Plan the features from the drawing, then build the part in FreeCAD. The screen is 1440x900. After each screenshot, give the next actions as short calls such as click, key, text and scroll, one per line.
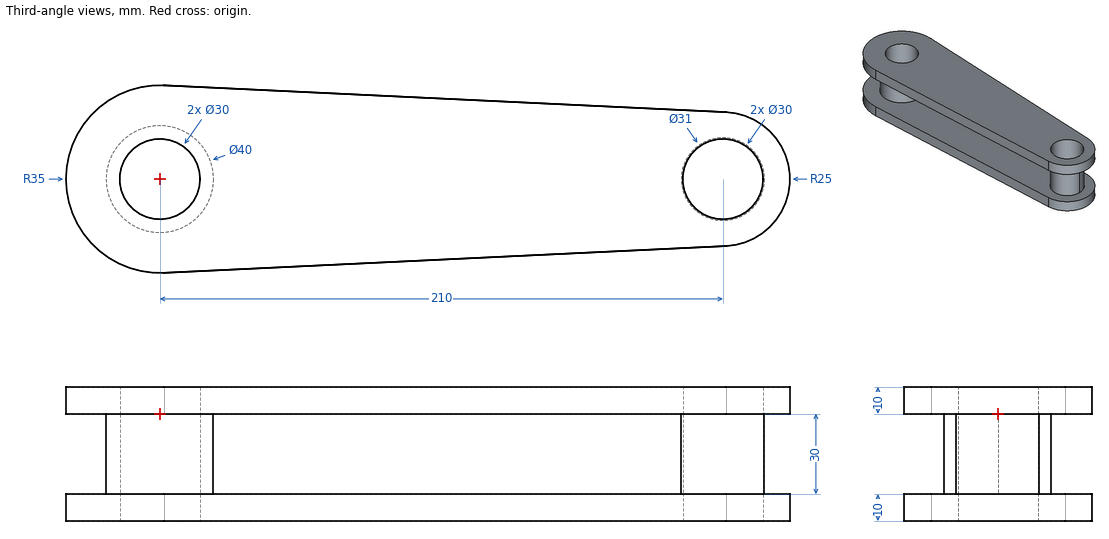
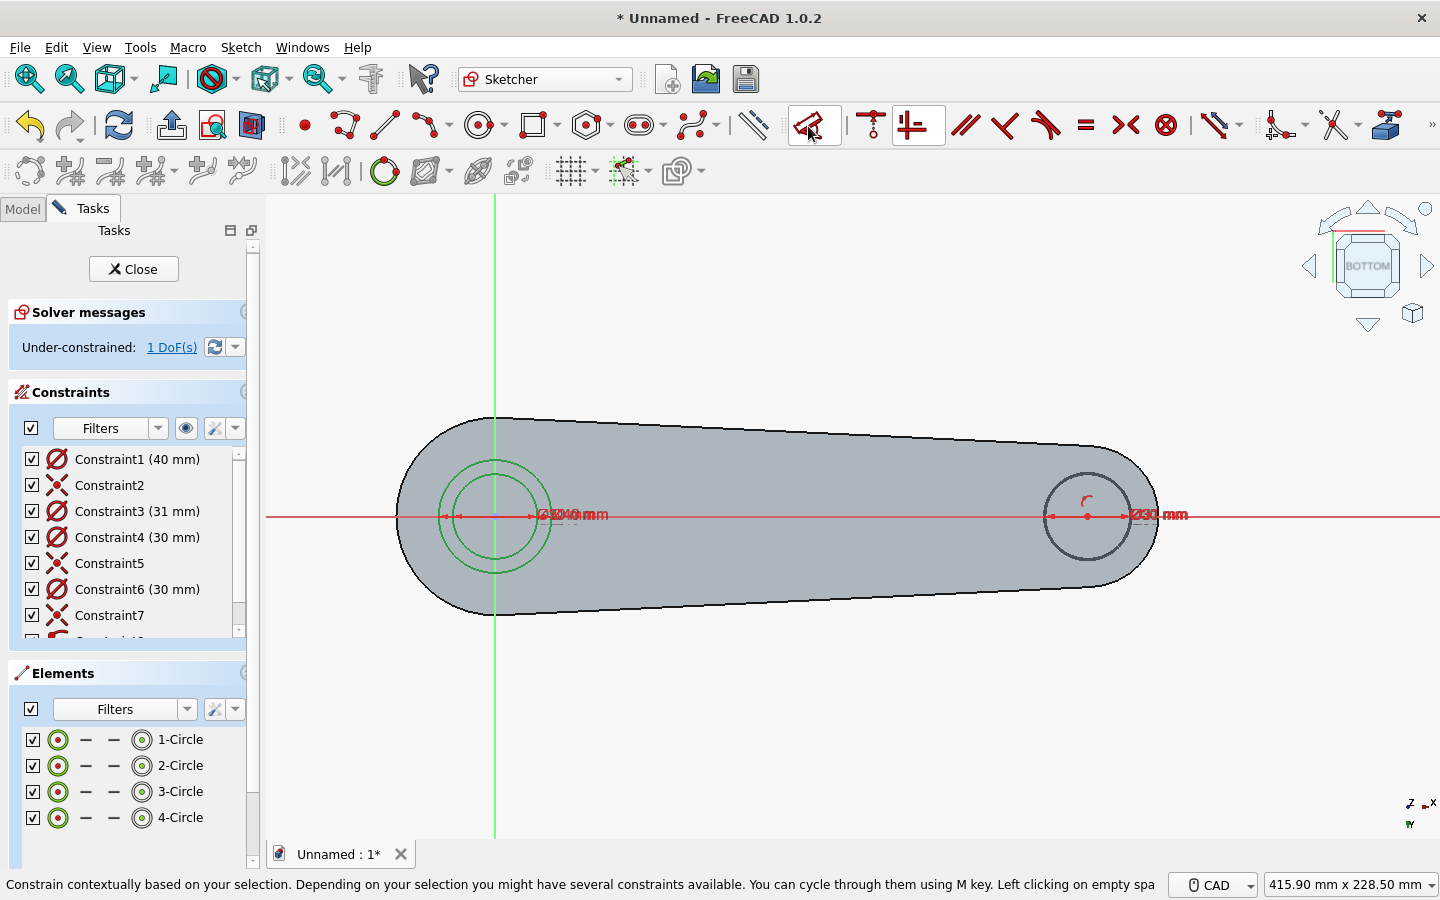
click(1088, 517)
click(791, 551)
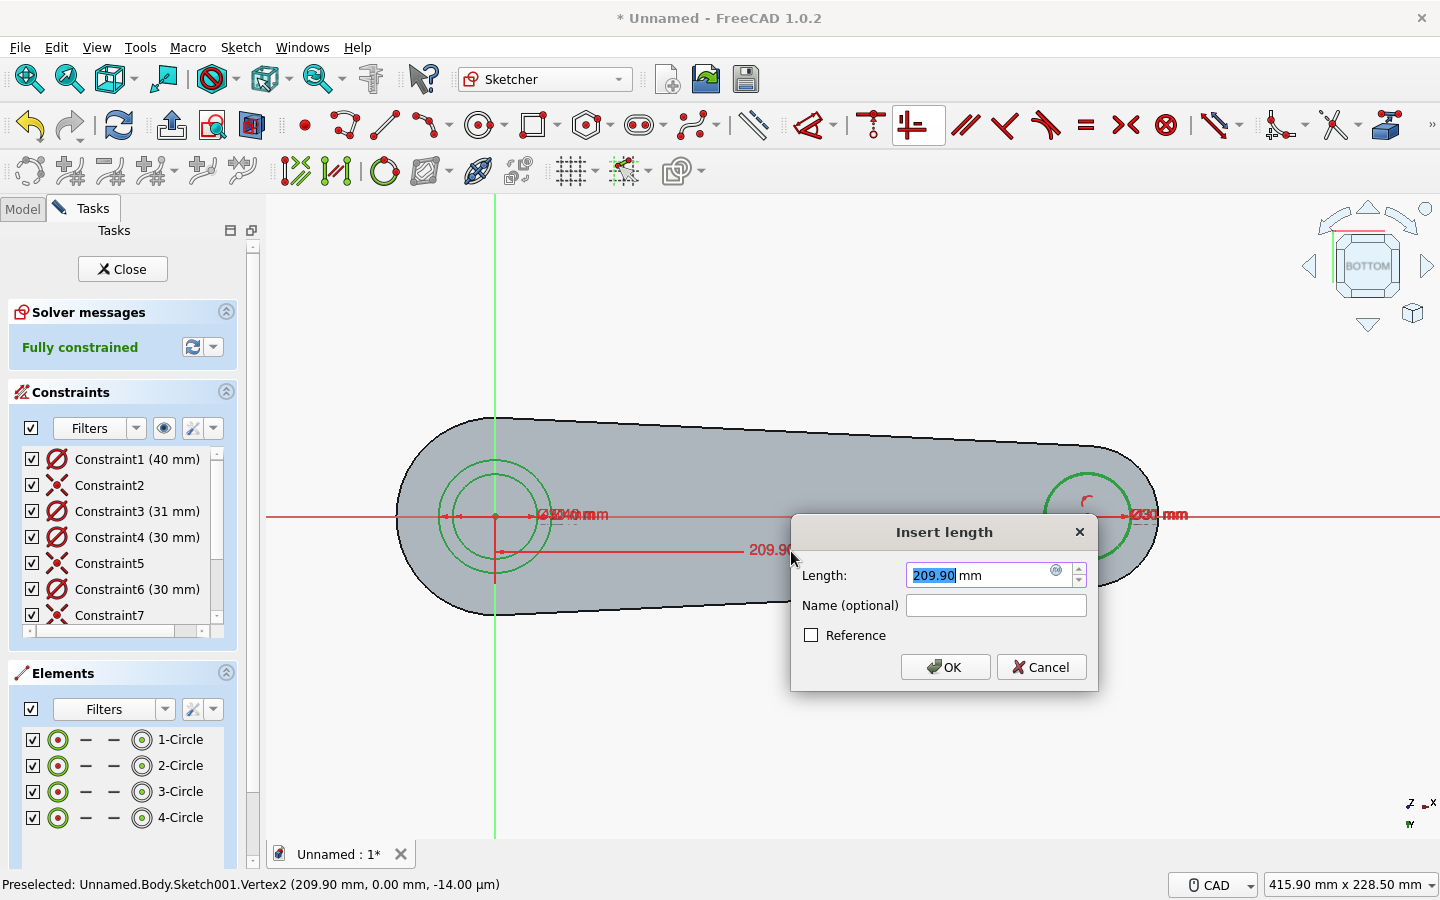
text(210)
key(Return)
key(Escape)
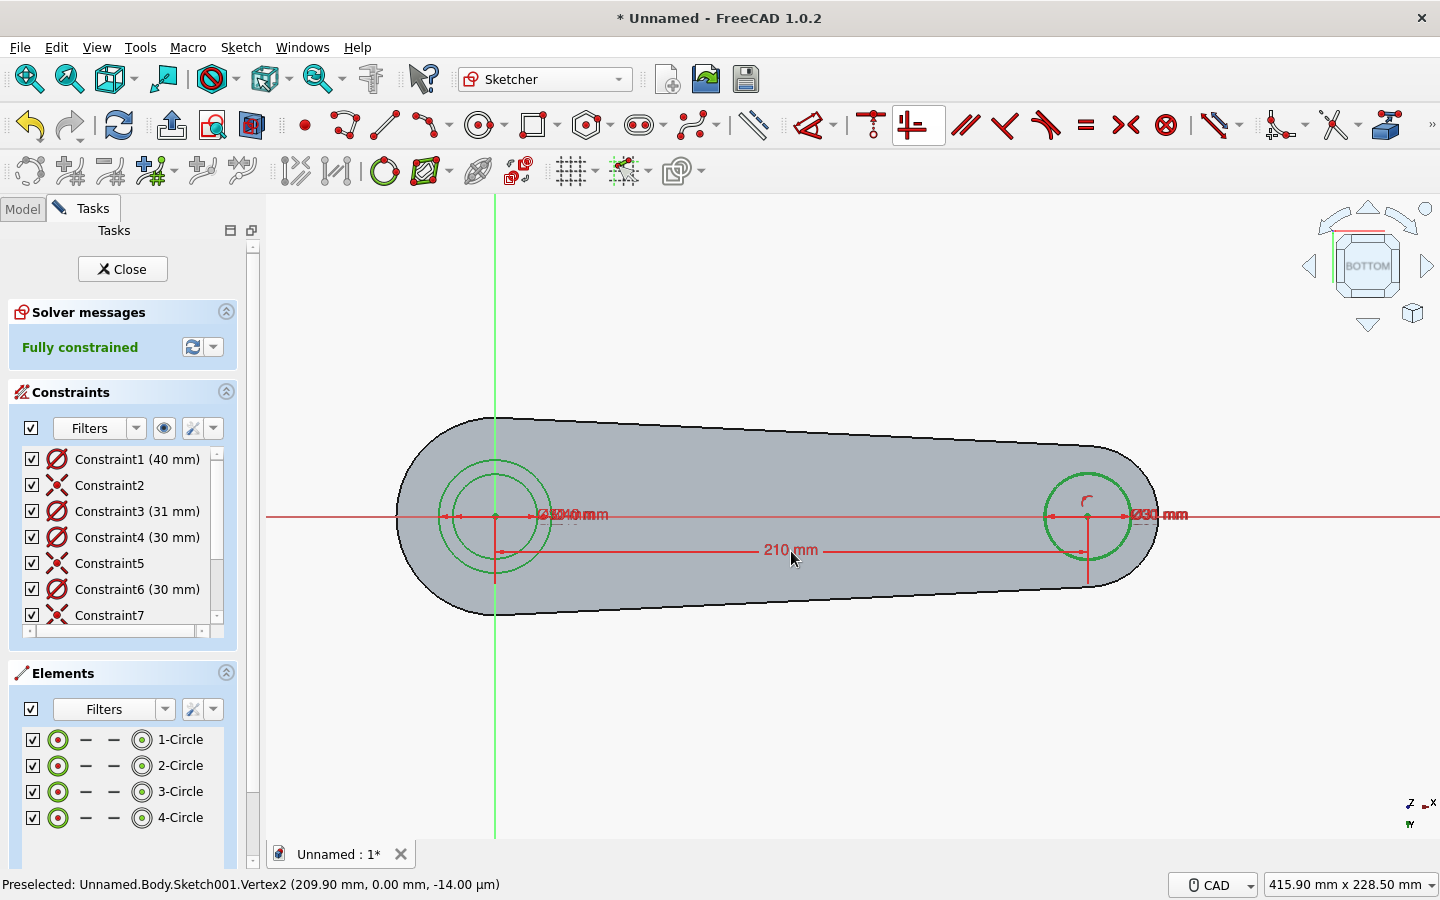
click(123, 269)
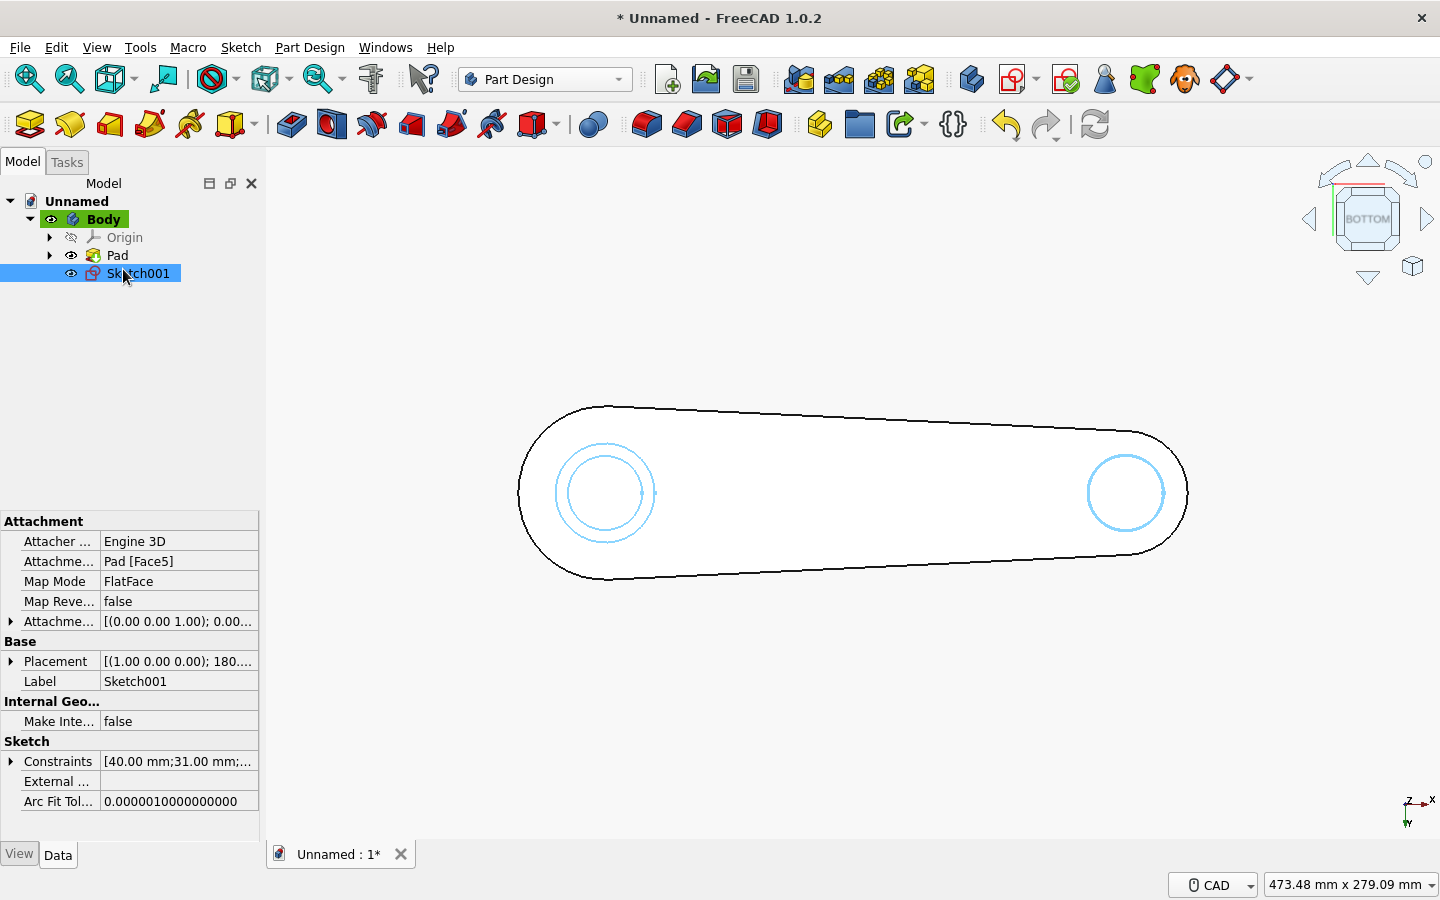
click(30, 124)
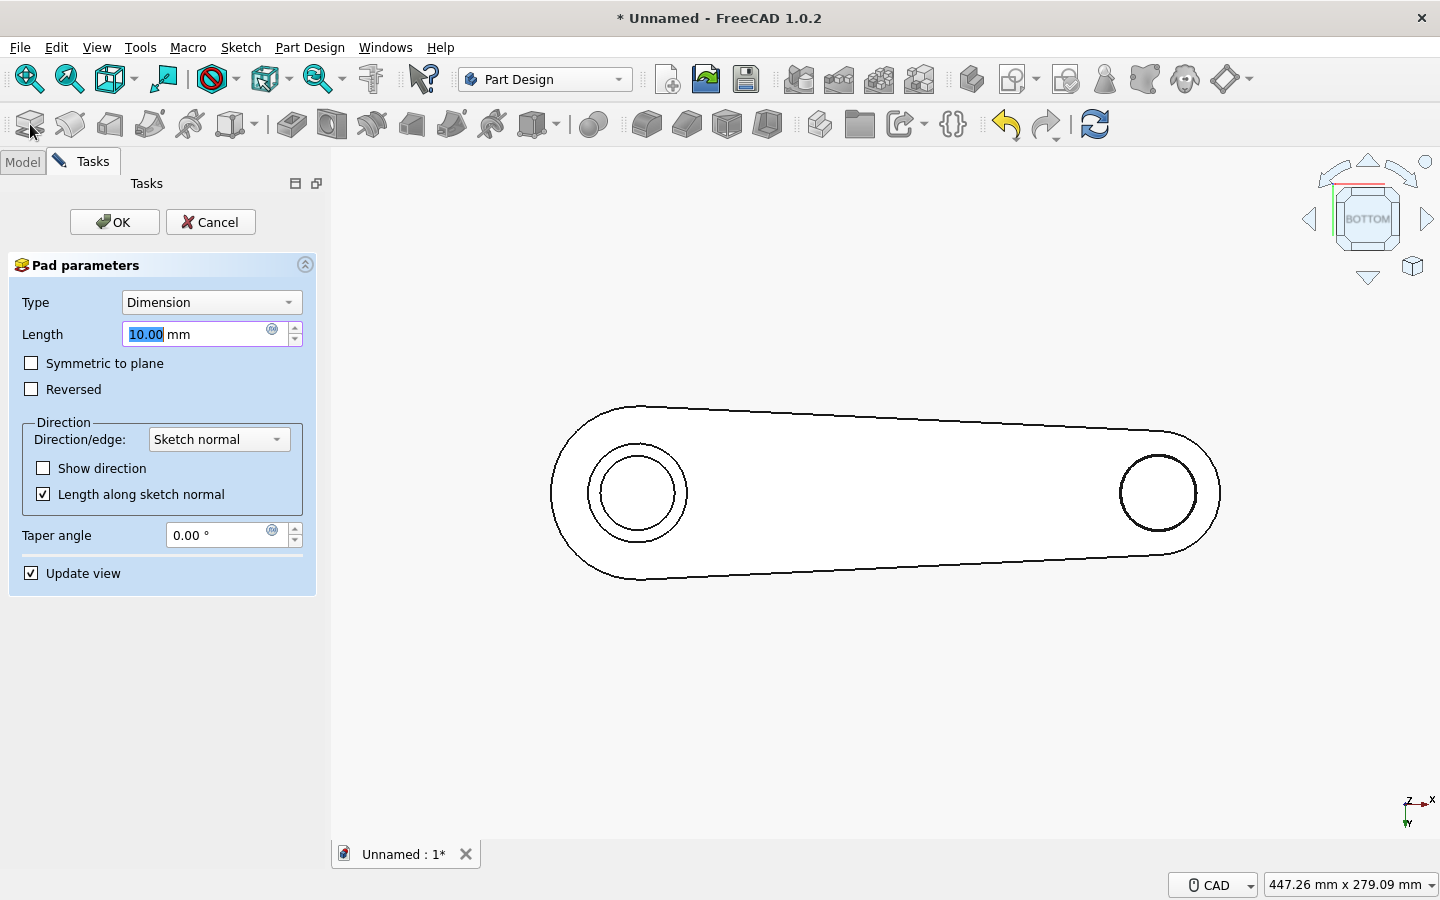
text(30)
key(Tab)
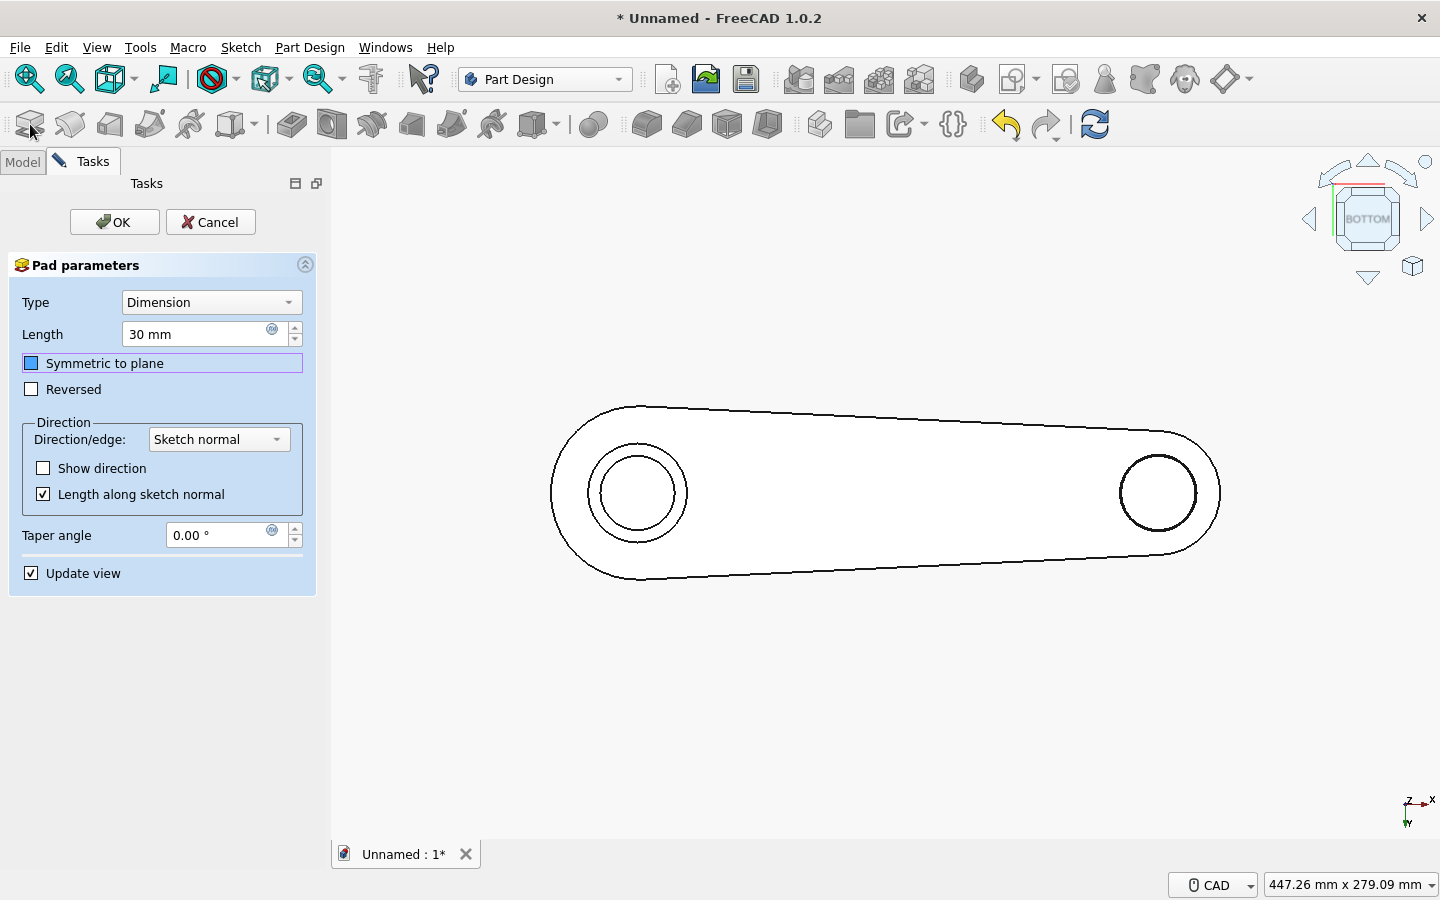
click(115, 222)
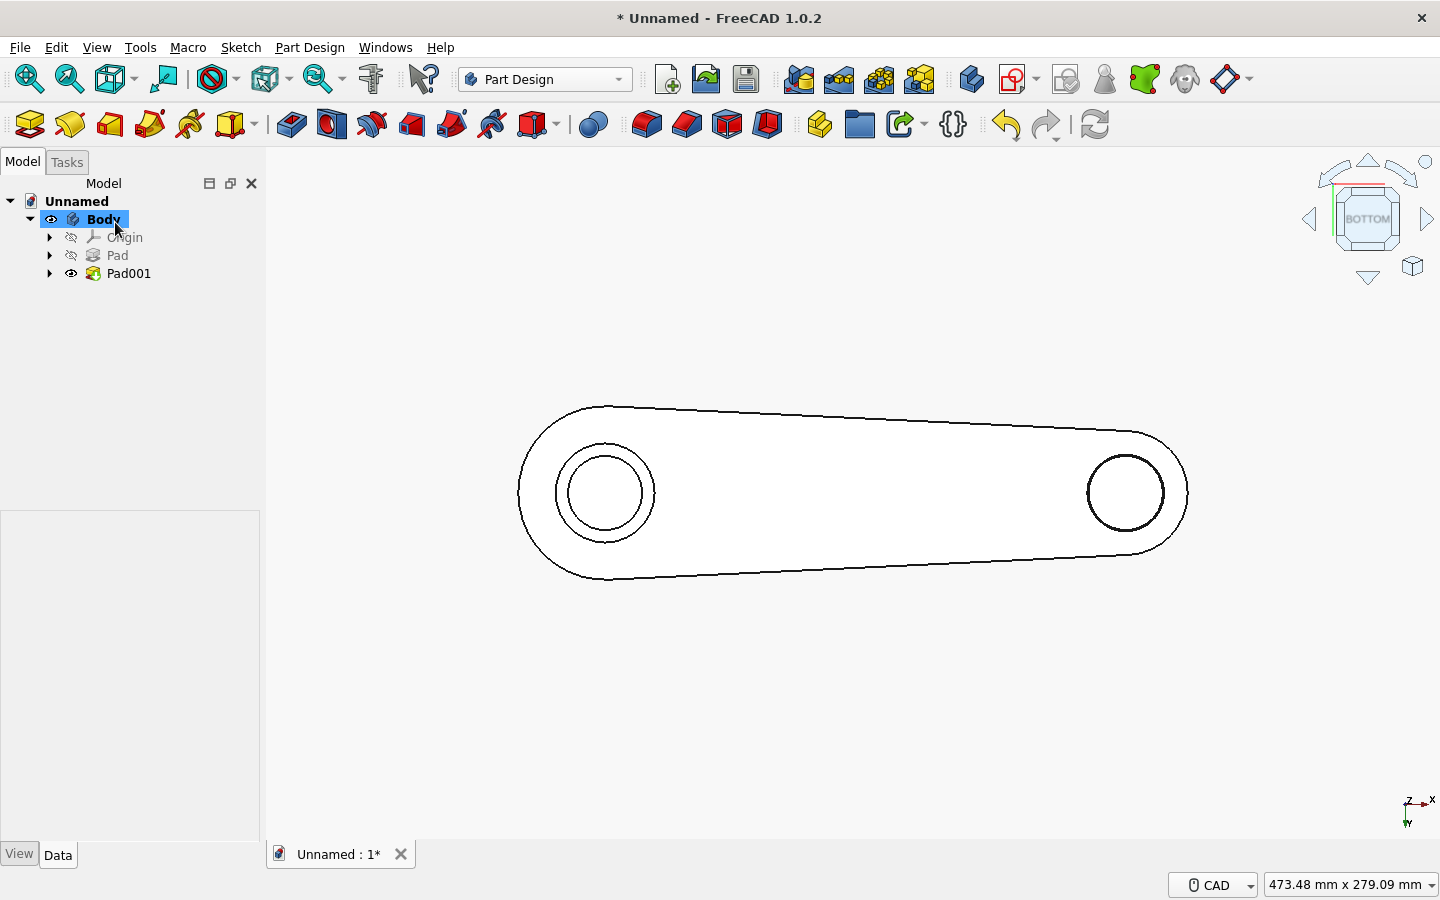
click(50, 237)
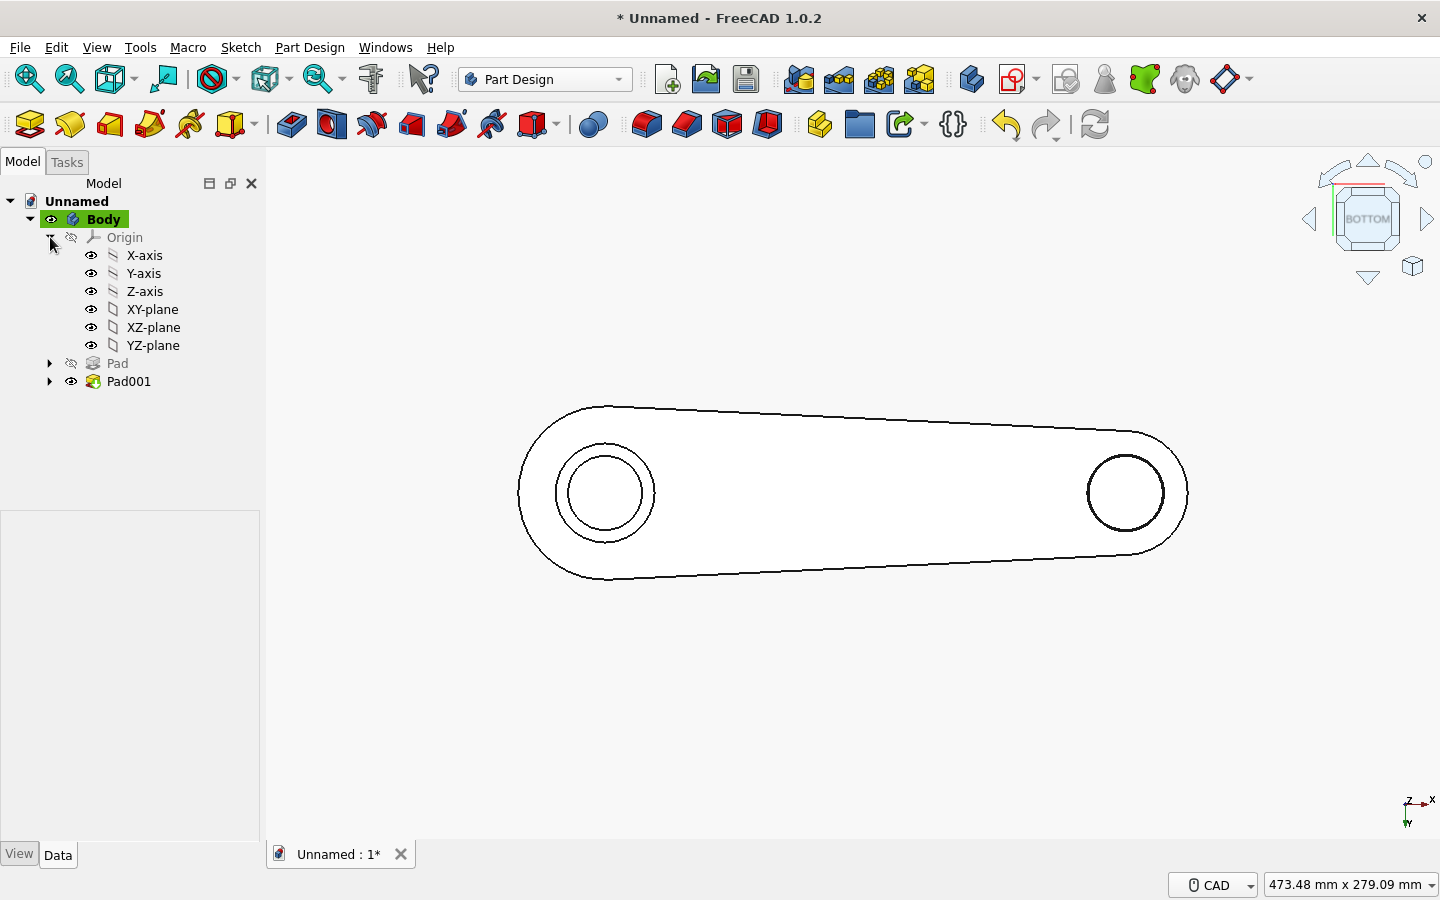
click(136, 309)